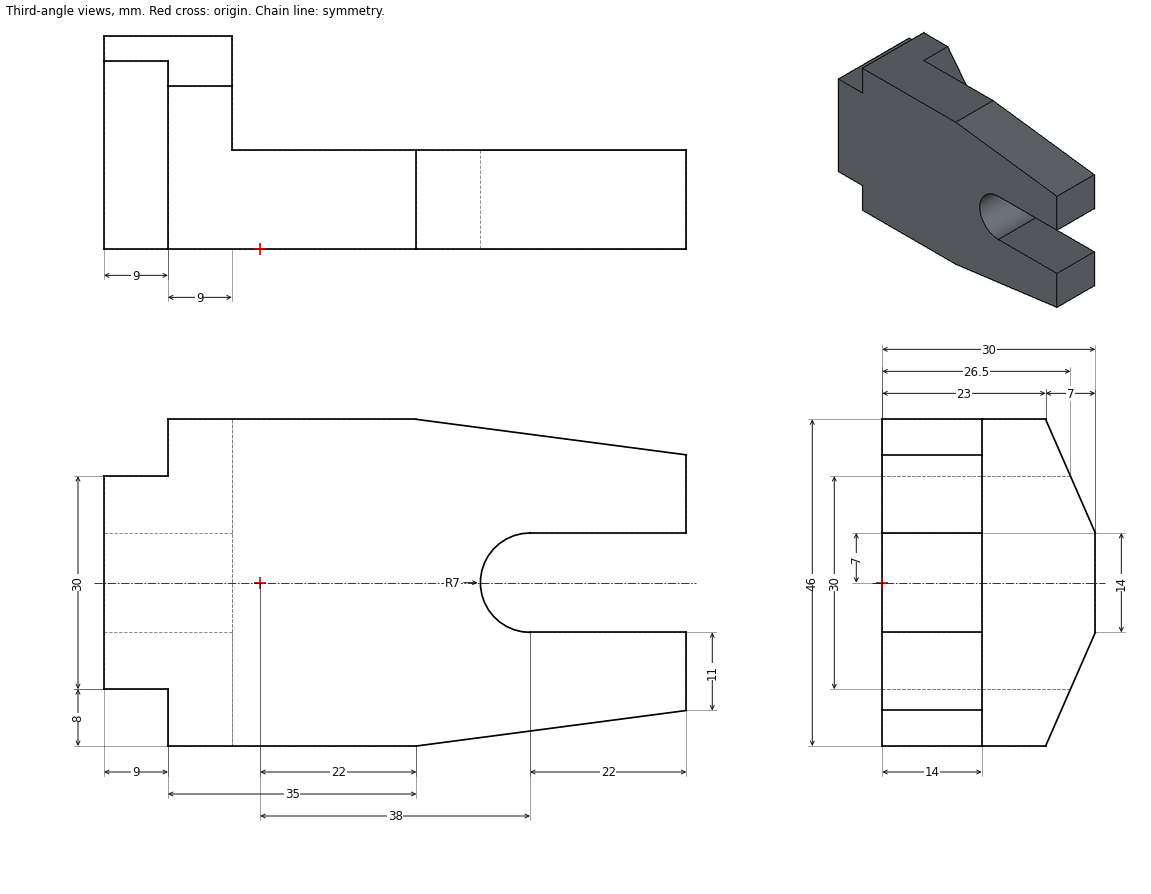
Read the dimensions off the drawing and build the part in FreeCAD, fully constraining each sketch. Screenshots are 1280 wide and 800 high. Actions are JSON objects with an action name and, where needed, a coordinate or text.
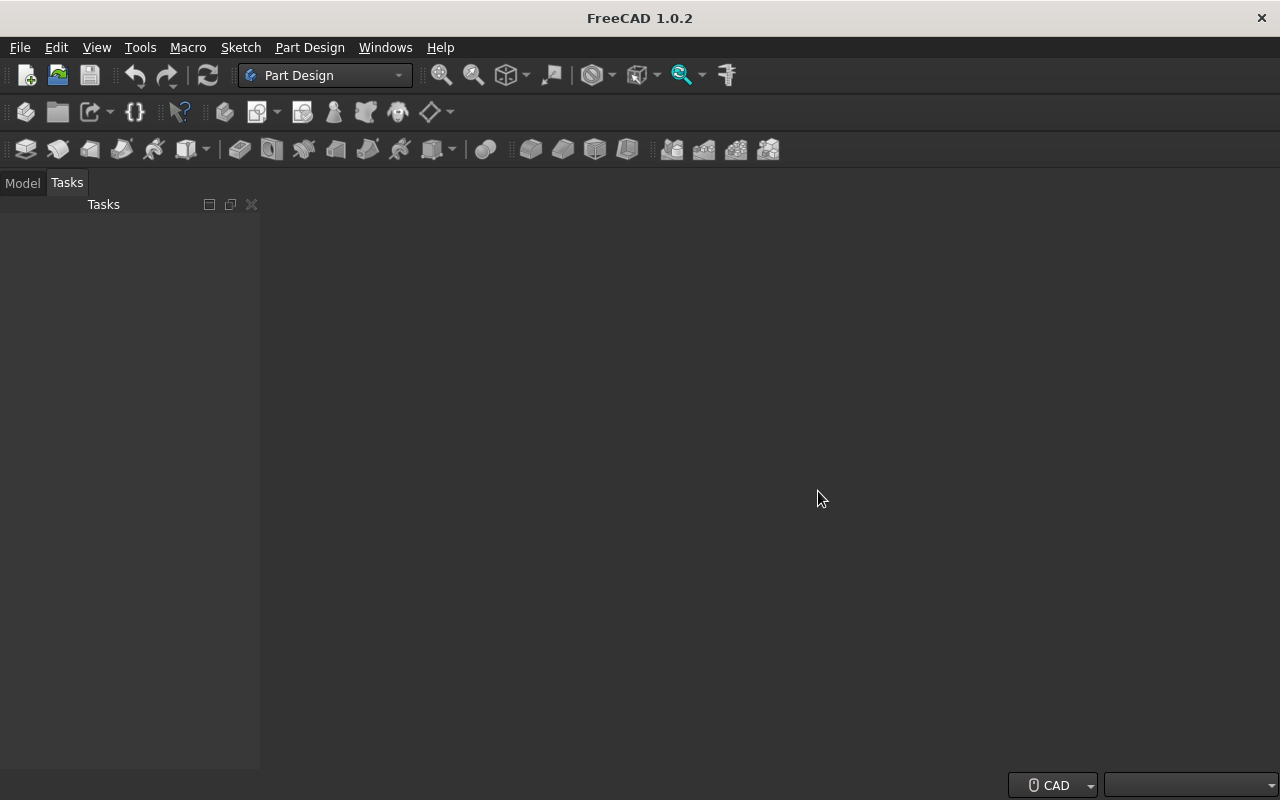
{"action": "left_click", "coordinate": [26, 76]}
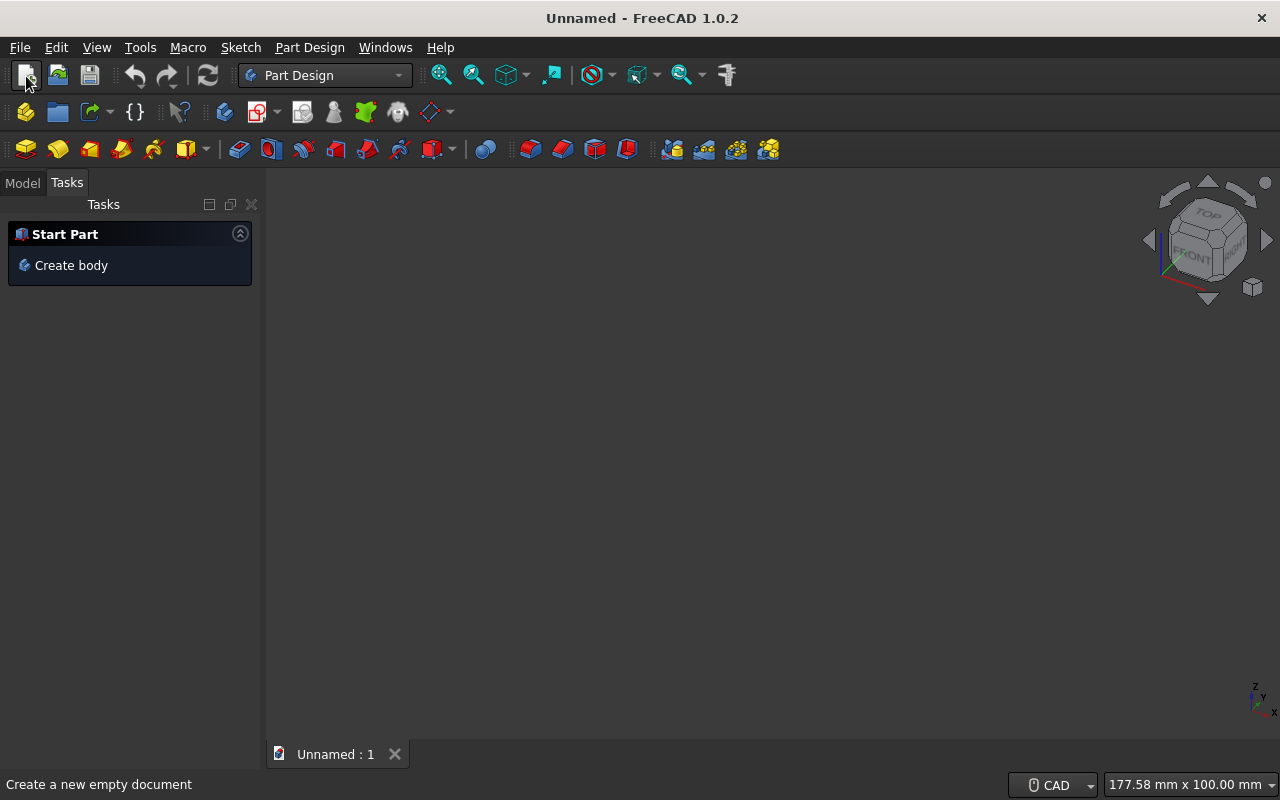
{"action": "left_click", "coordinate": [258, 112]}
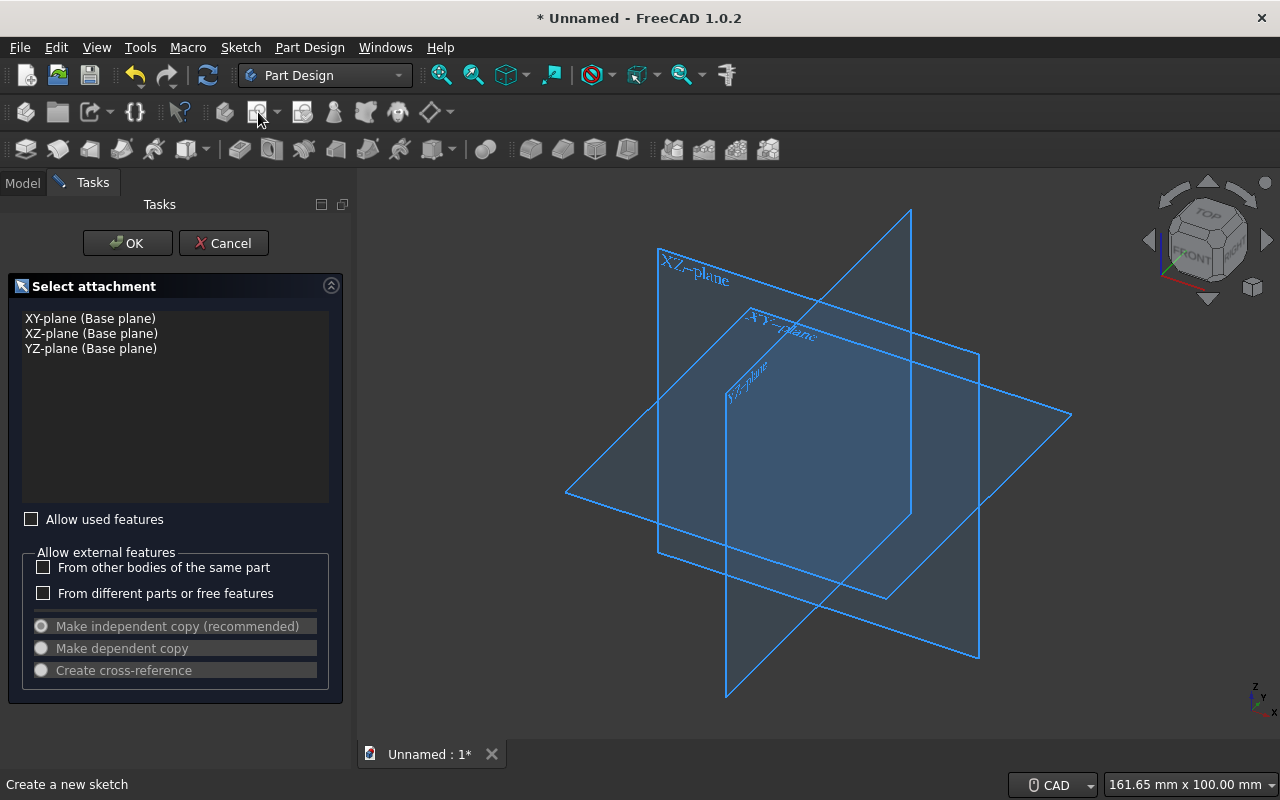
{"action": "left_click", "coordinate": [82, 334]}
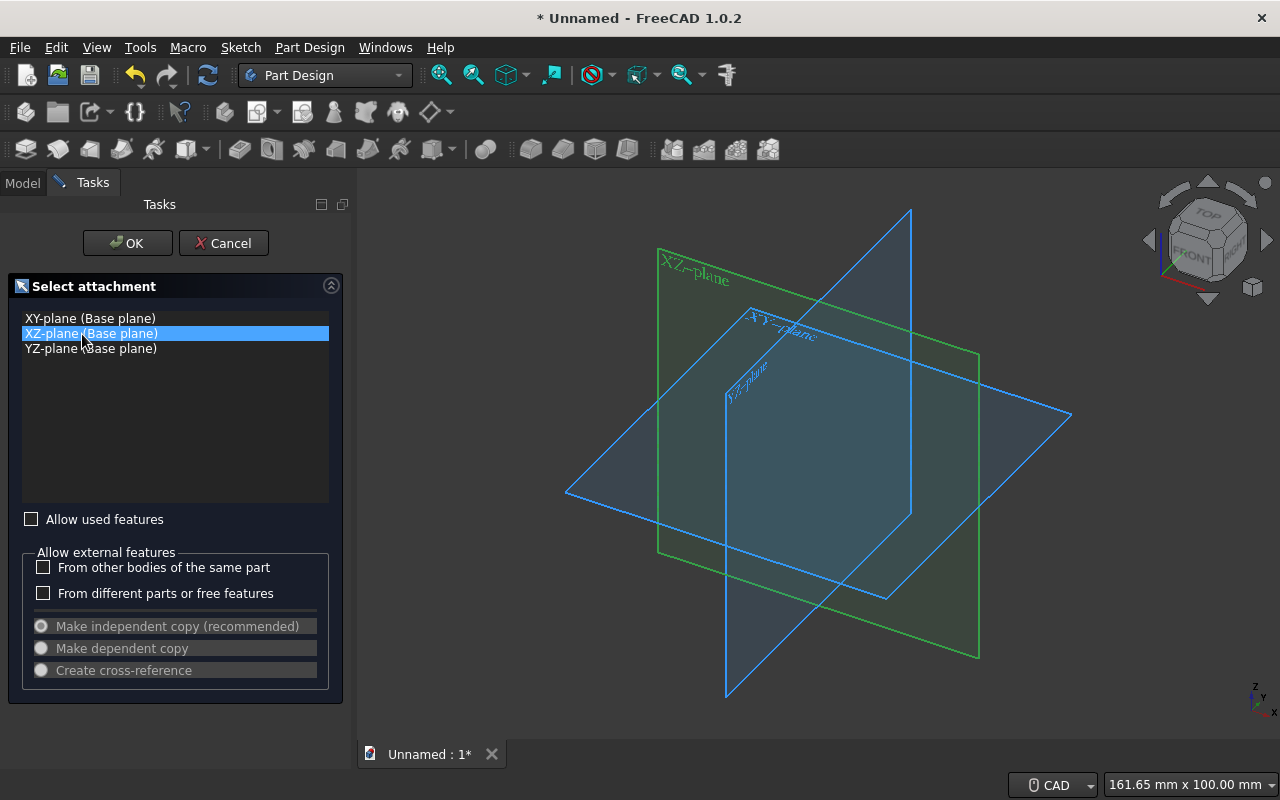
{"action": "left_click", "coordinate": [128, 243]}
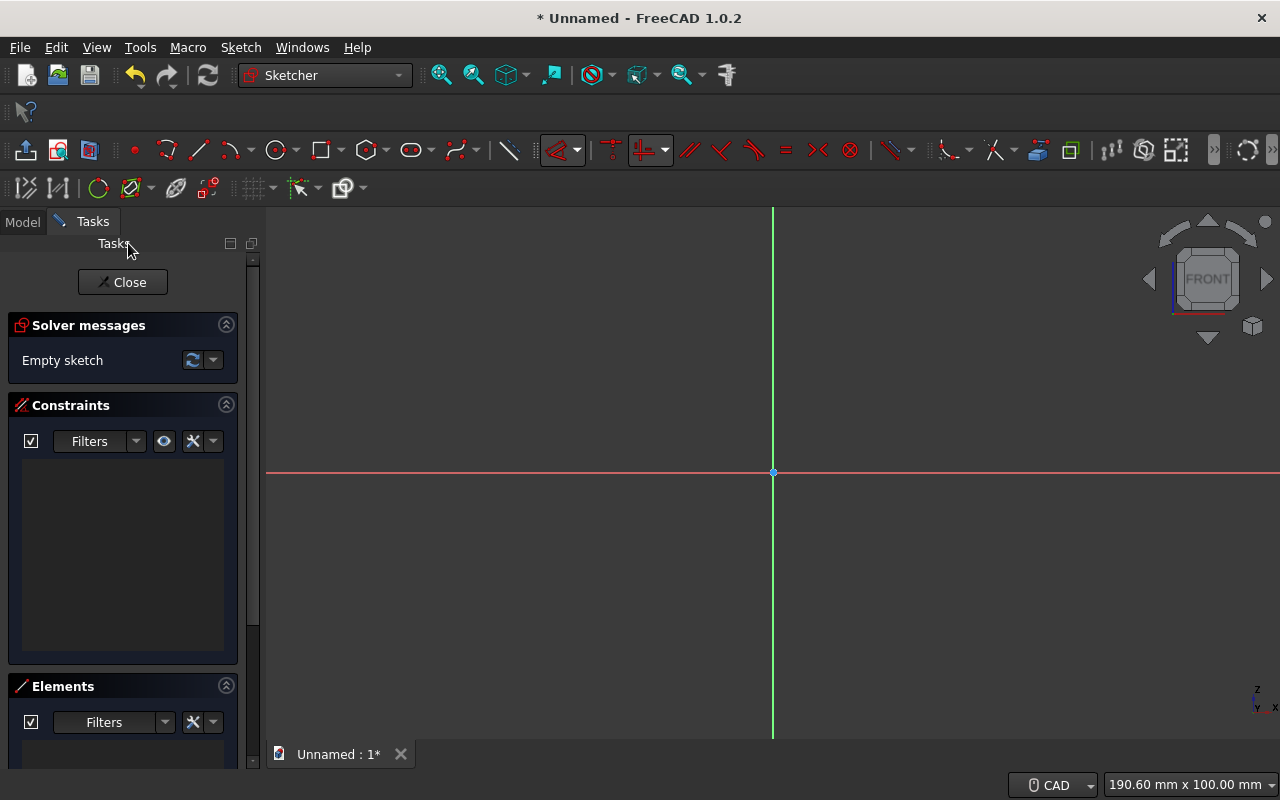
{"action": "scroll", "coordinate": [1115, 473], "scroll_direction": "up", "scroll_amount": 1}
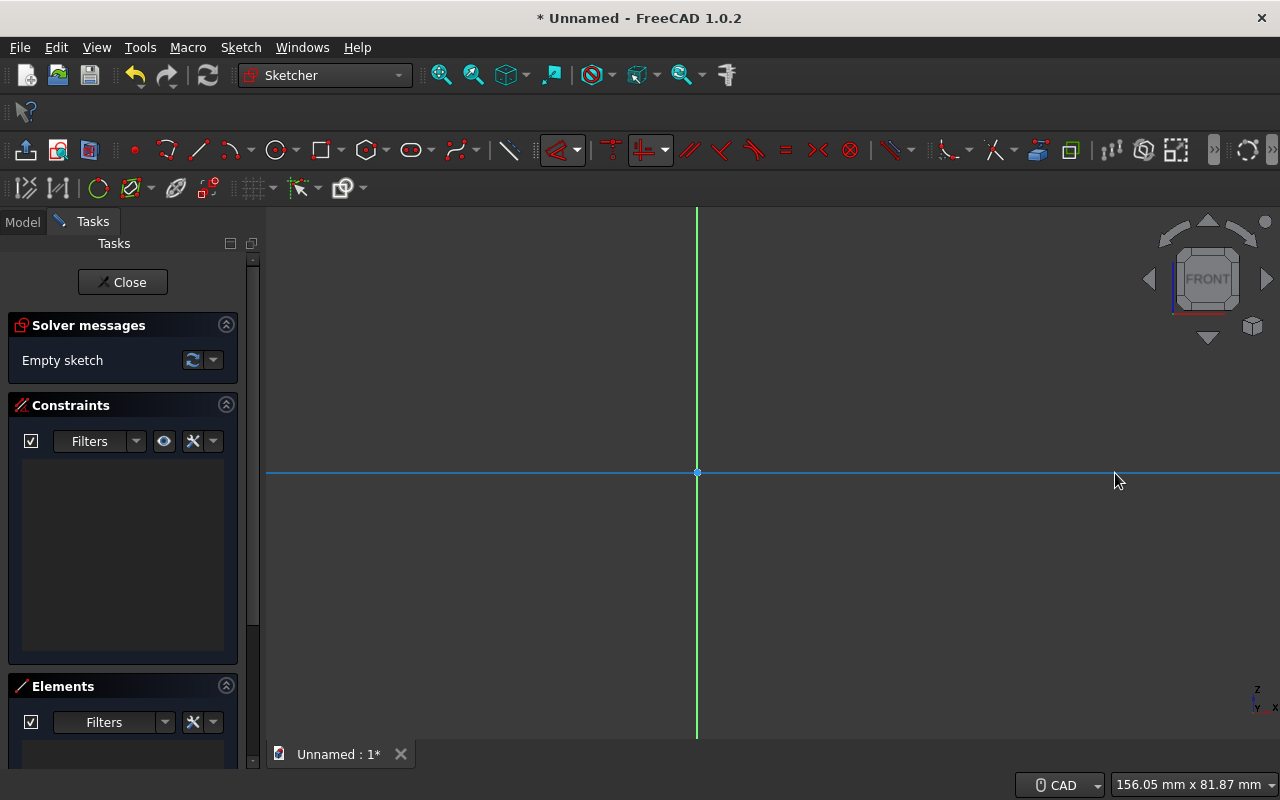
{"action": "left_click", "coordinate": [168, 150]}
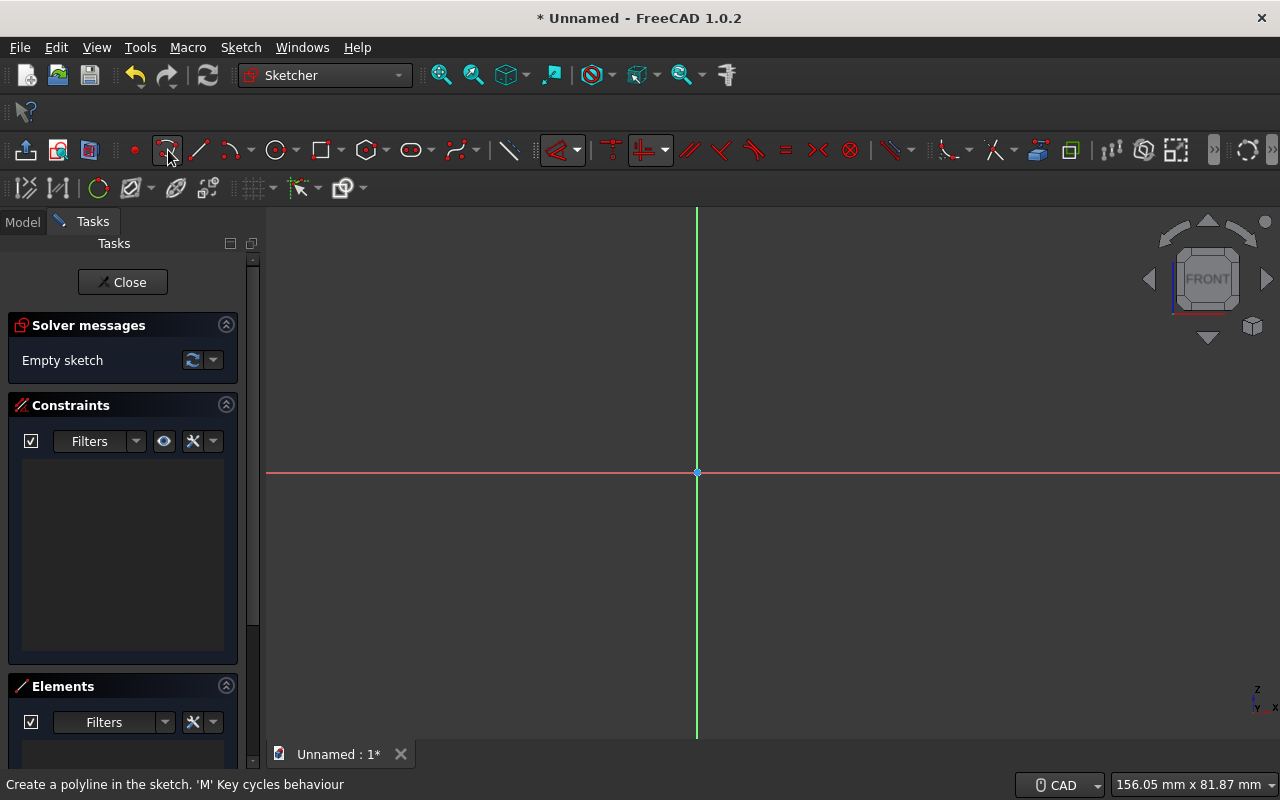
{"action": "left_click", "coordinate": [944, 518]}
{"action": "left_click", "coordinate": [1087, 518]}
{"action": "left_click", "coordinate": [1087, 590]}
{"action": "left_click", "coordinate": [840, 622]}
{"action": "left_click", "coordinate": [613, 622]}
{"action": "left_click", "coordinate": [613, 570]}
{"action": "left_click", "coordinate": [554, 570]}
{"action": "left_click", "coordinate": [554, 375]}
{"action": "left_click", "coordinate": [613, 375]}
{"action": "left_click", "coordinate": [613, 323]}
{"action": "left_click", "coordinate": [840, 323]}
{"action": "left_click", "coordinate": [1087, 356]}
{"action": "left_click", "coordinate": [1087, 427]}
{"action": "left_click", "coordinate": [944, 427]}
{"action": "right_click", "coordinate": [944, 427]}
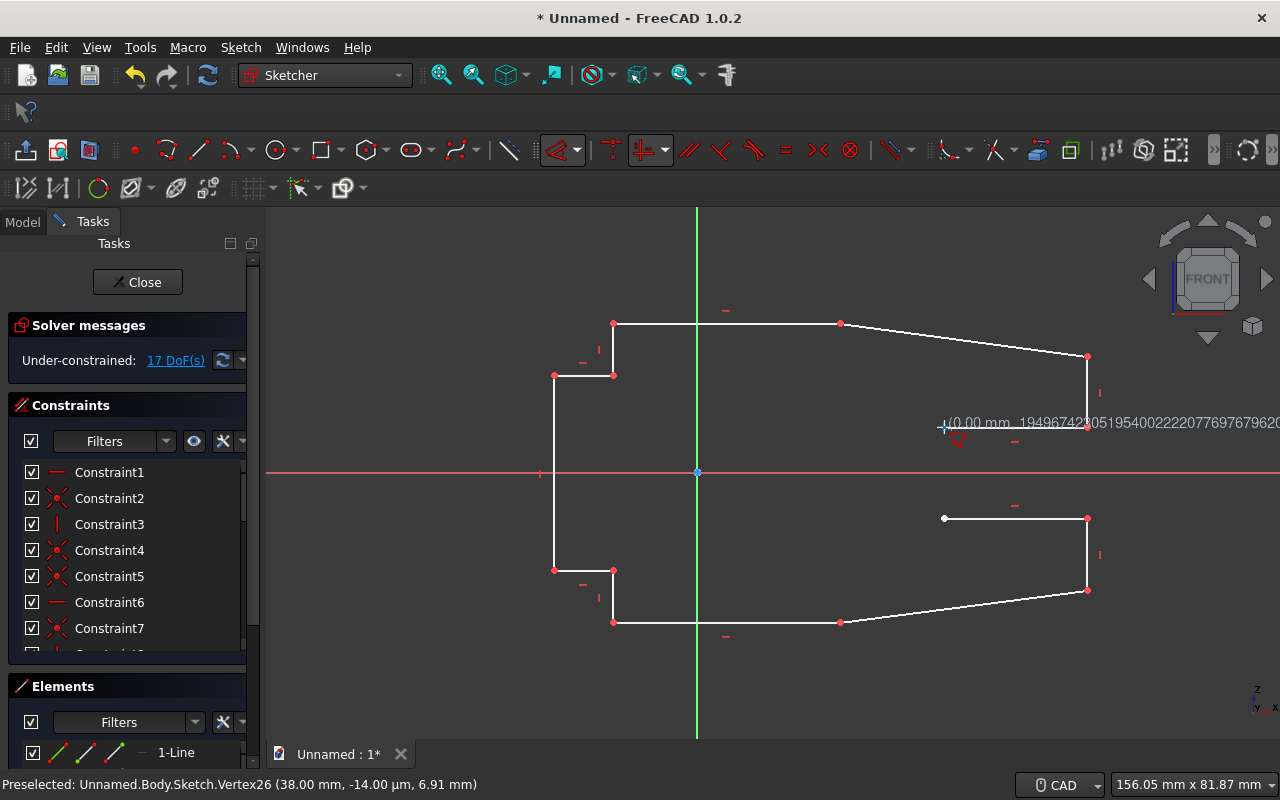
{"action": "key", "text": "g 3 a"}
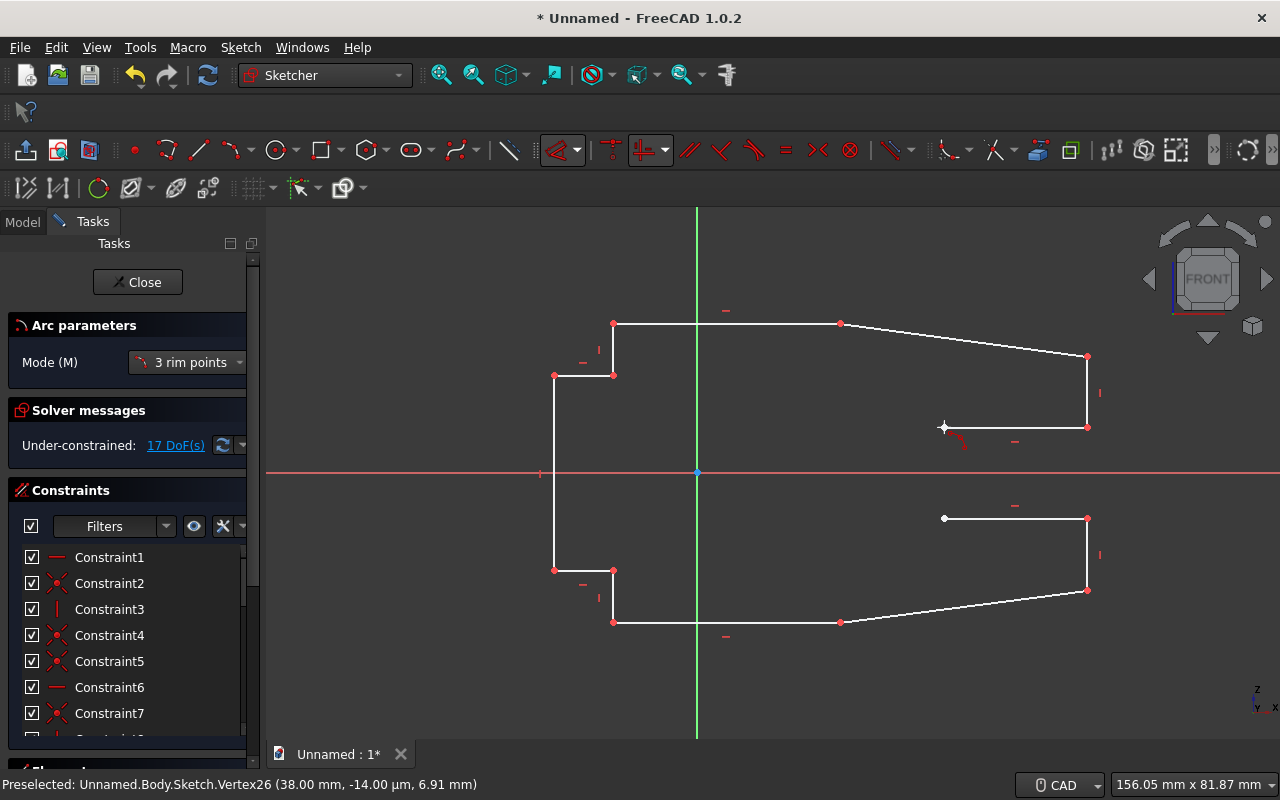
{"action": "left_click", "coordinate": [944, 428]}
{"action": "left_click", "coordinate": [944, 519]}
{"action": "left_click", "coordinate": [901, 459]}
{"action": "key", "text": "Escape"}